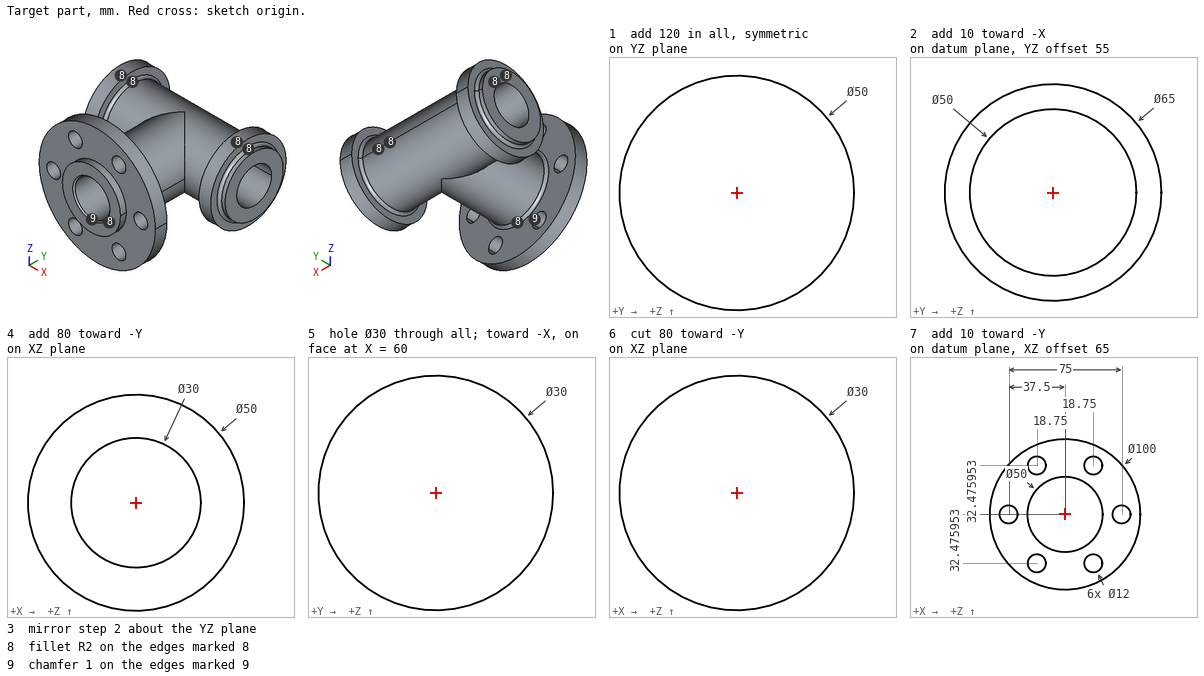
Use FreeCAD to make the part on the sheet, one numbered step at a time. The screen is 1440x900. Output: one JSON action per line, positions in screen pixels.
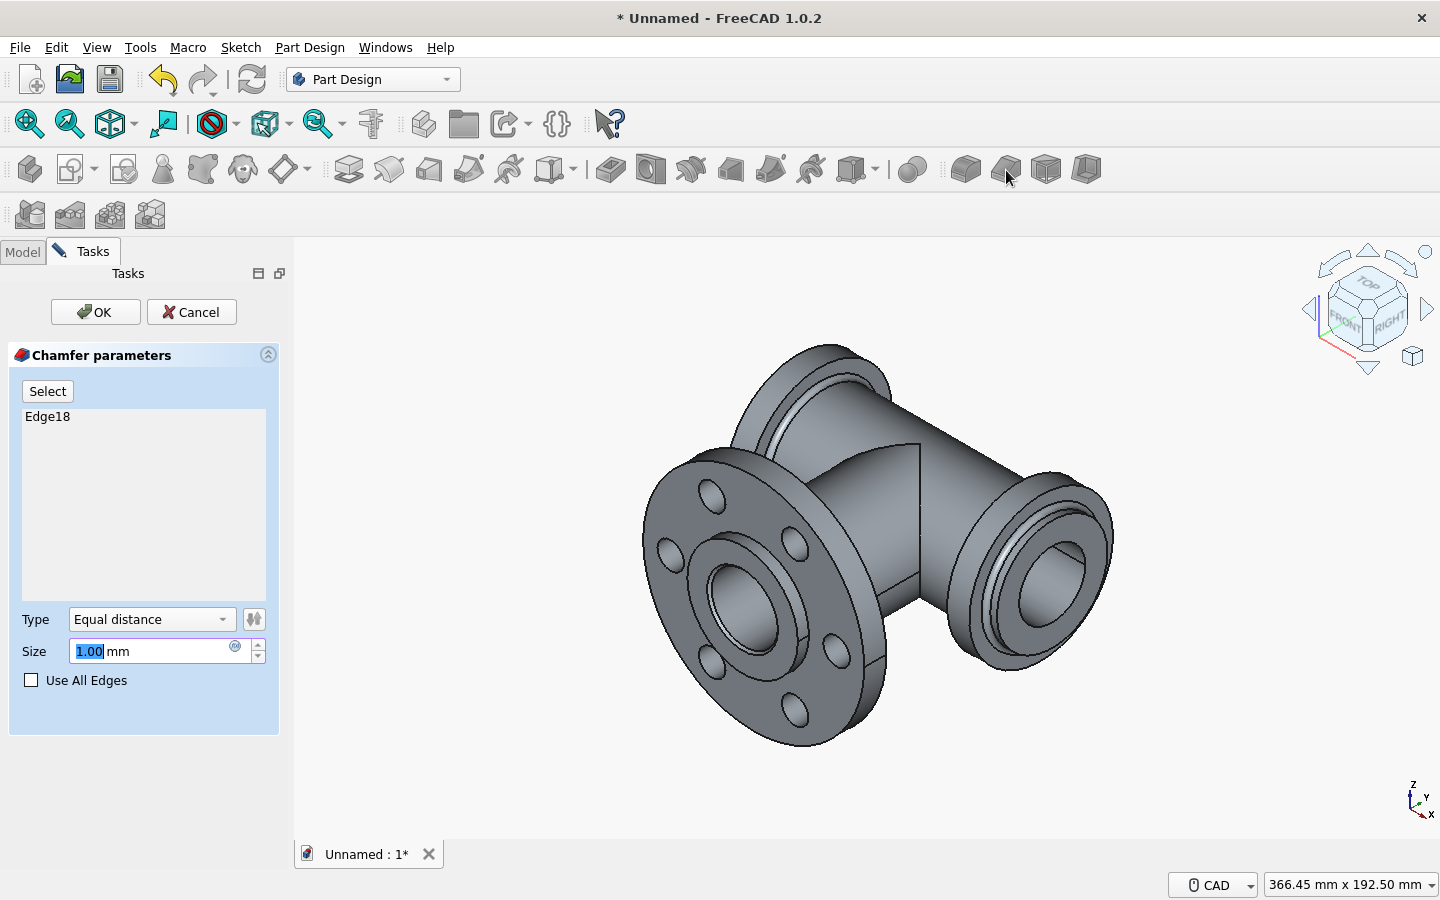
{"action": "type", "text": "1"}
{"action": "key", "text": "Tab"}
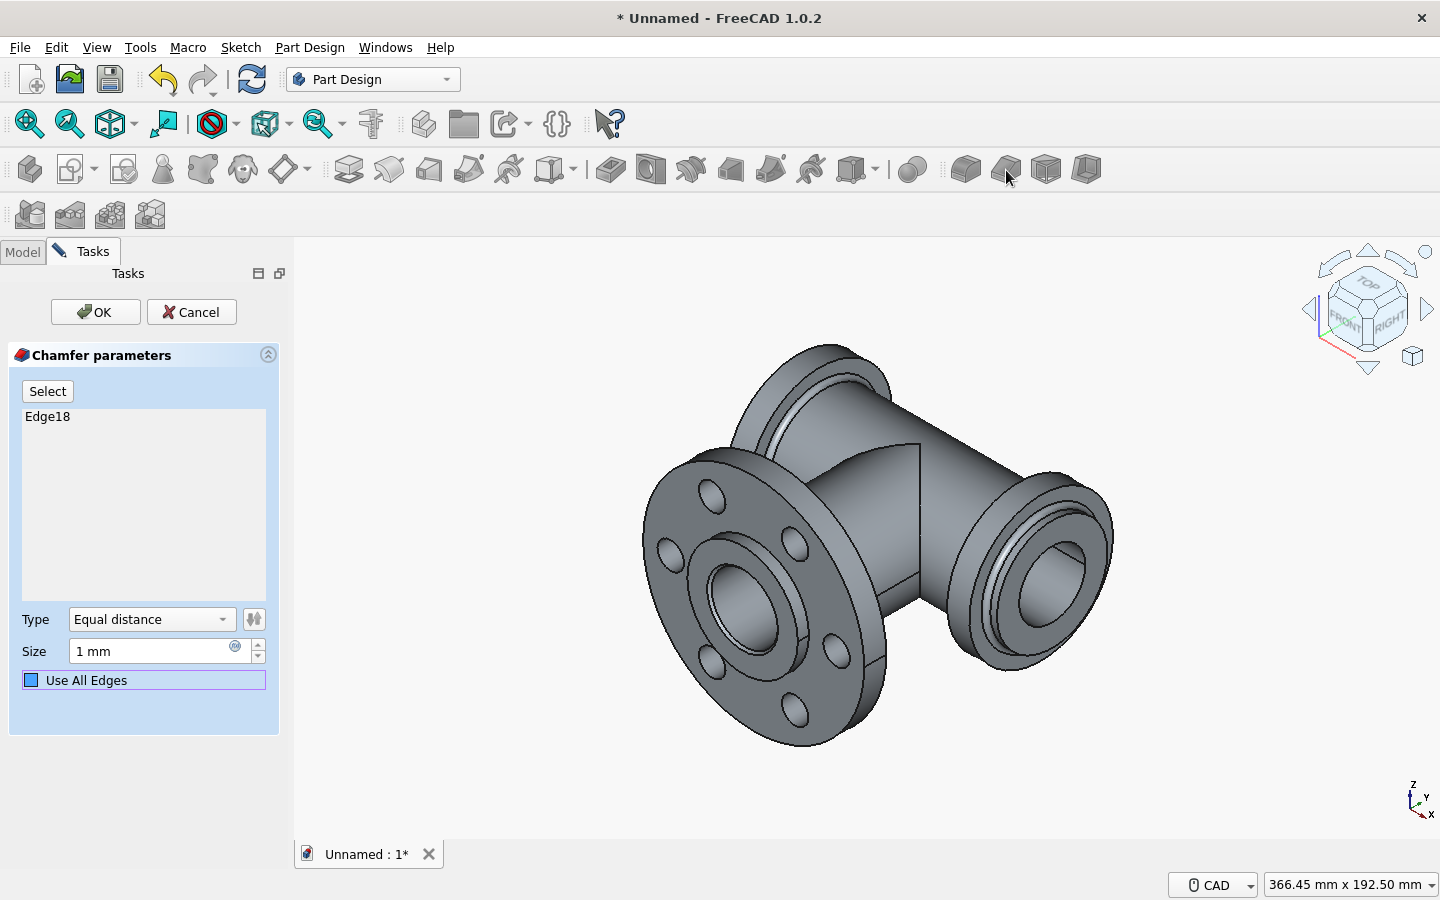
{"action": "left_click", "coordinate": [96, 312]}